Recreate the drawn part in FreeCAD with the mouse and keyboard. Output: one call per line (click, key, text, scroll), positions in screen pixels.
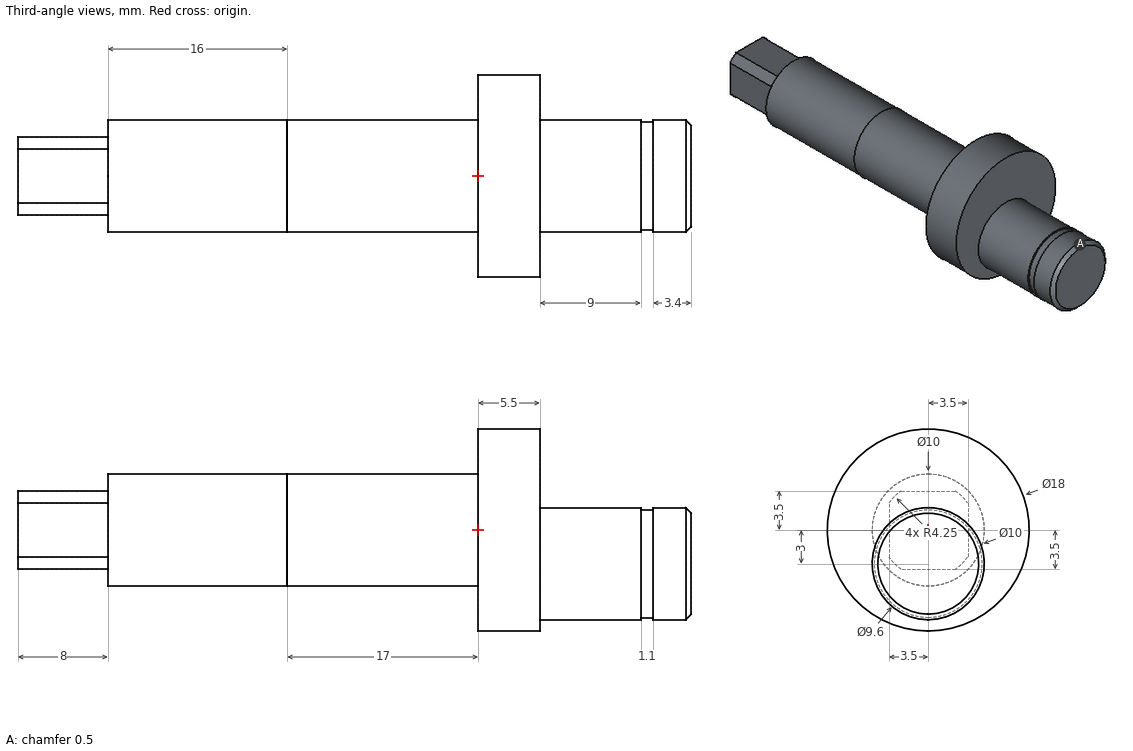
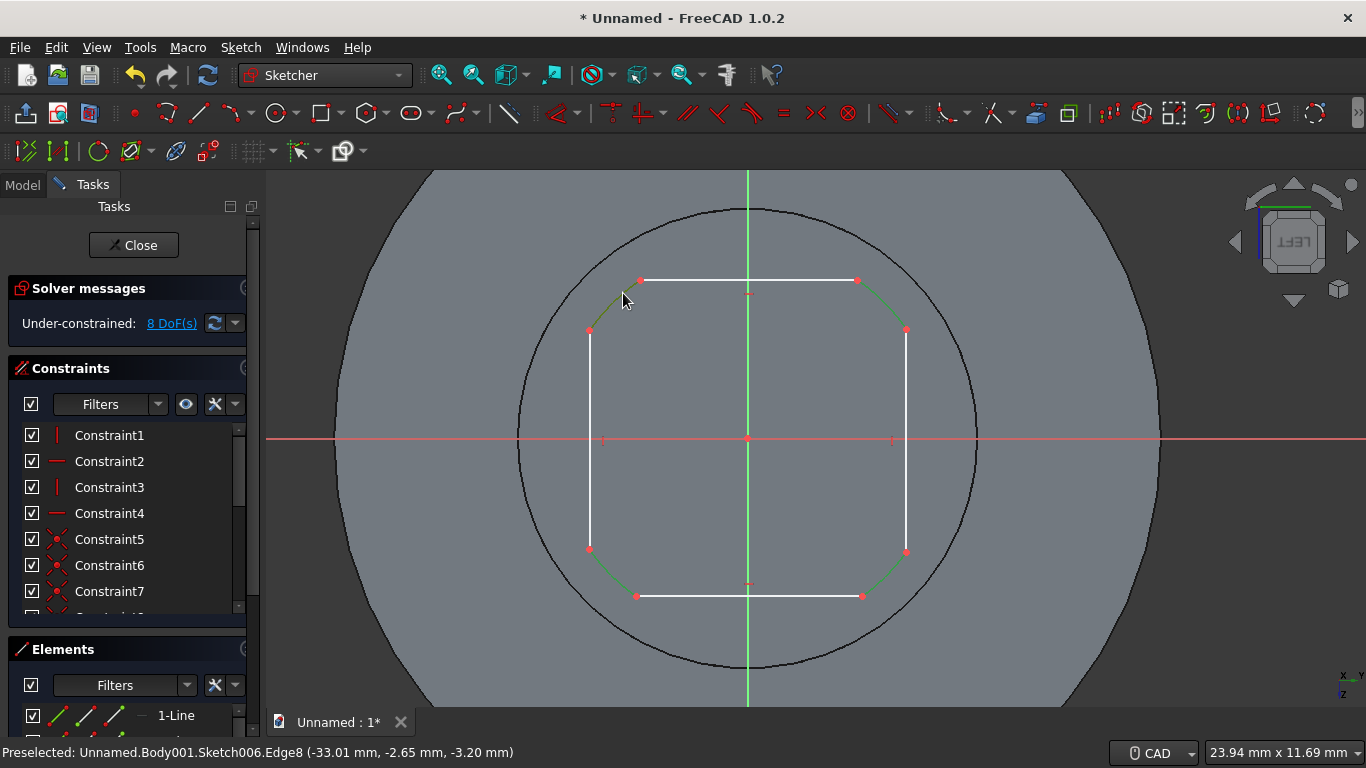
click(784, 114)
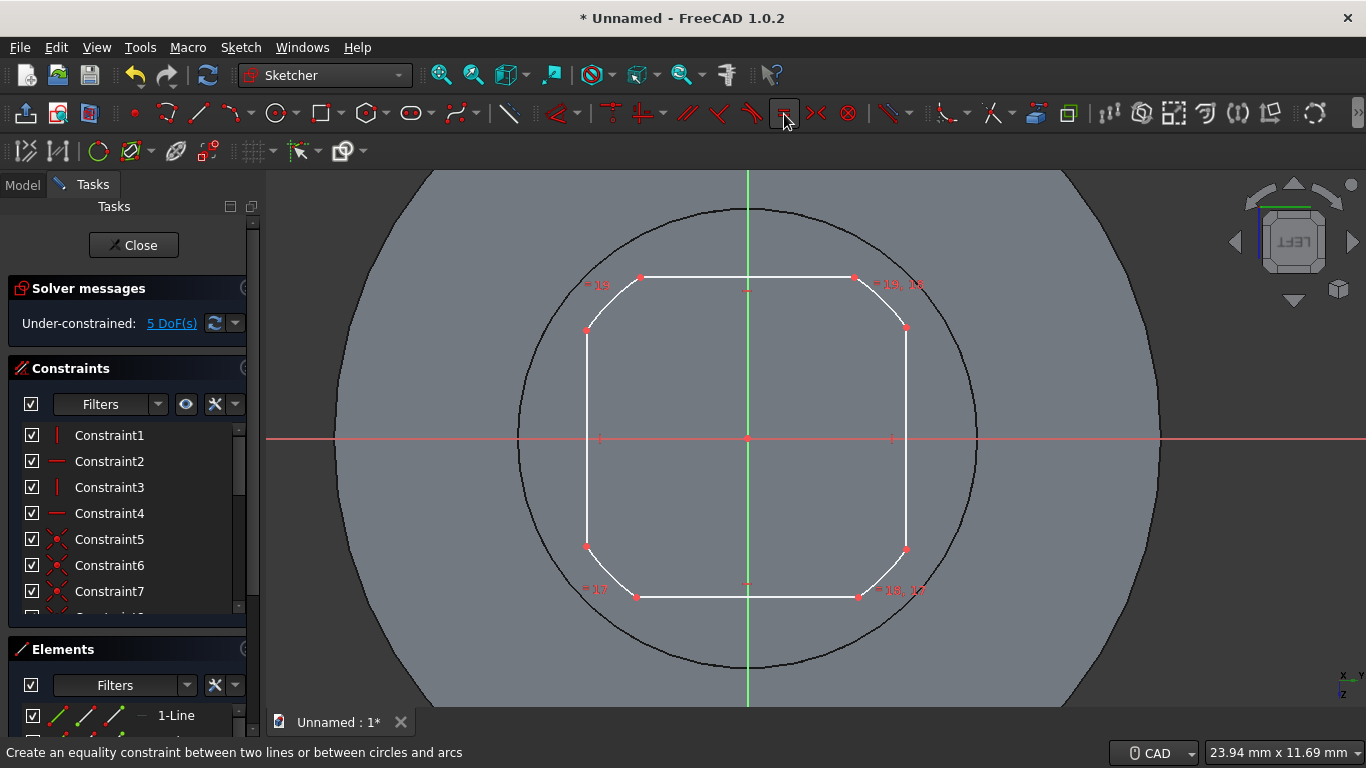
key(d)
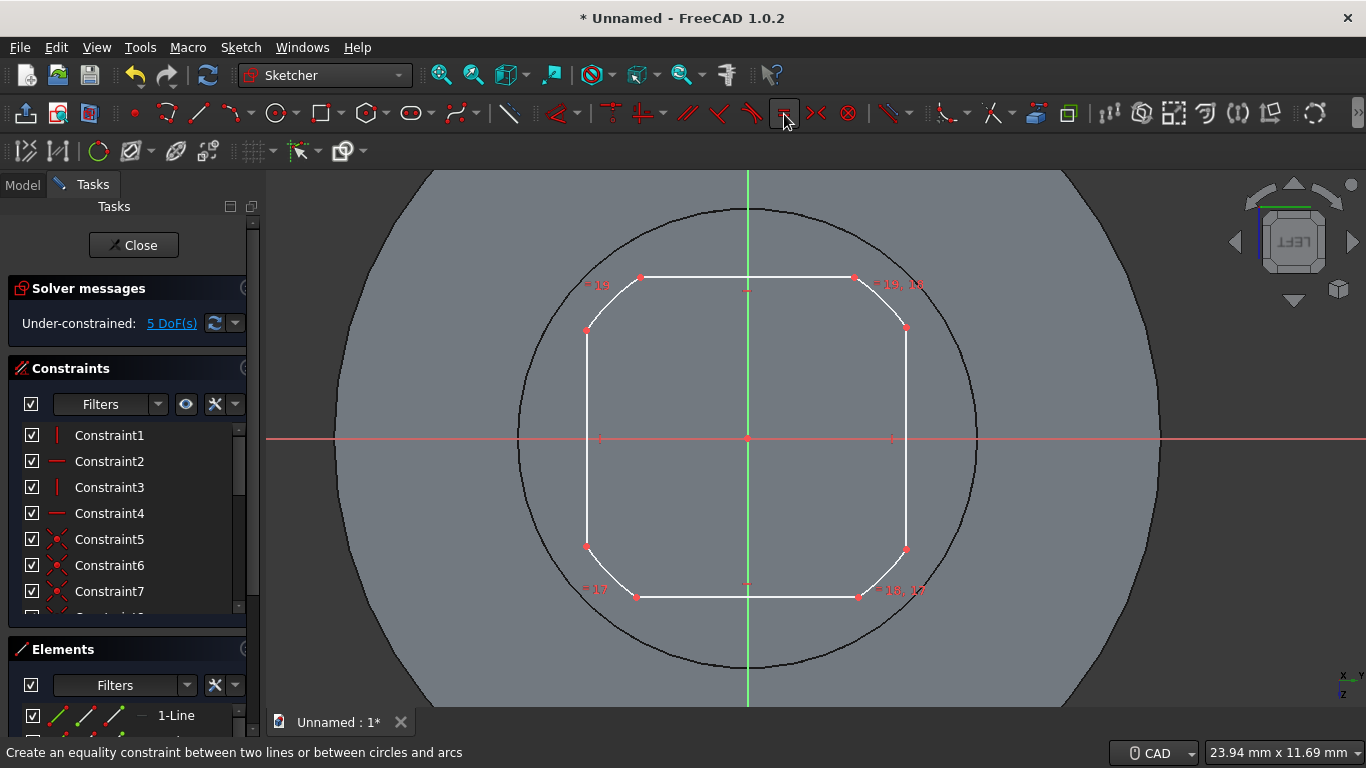
click(600, 563)
click(576, 584)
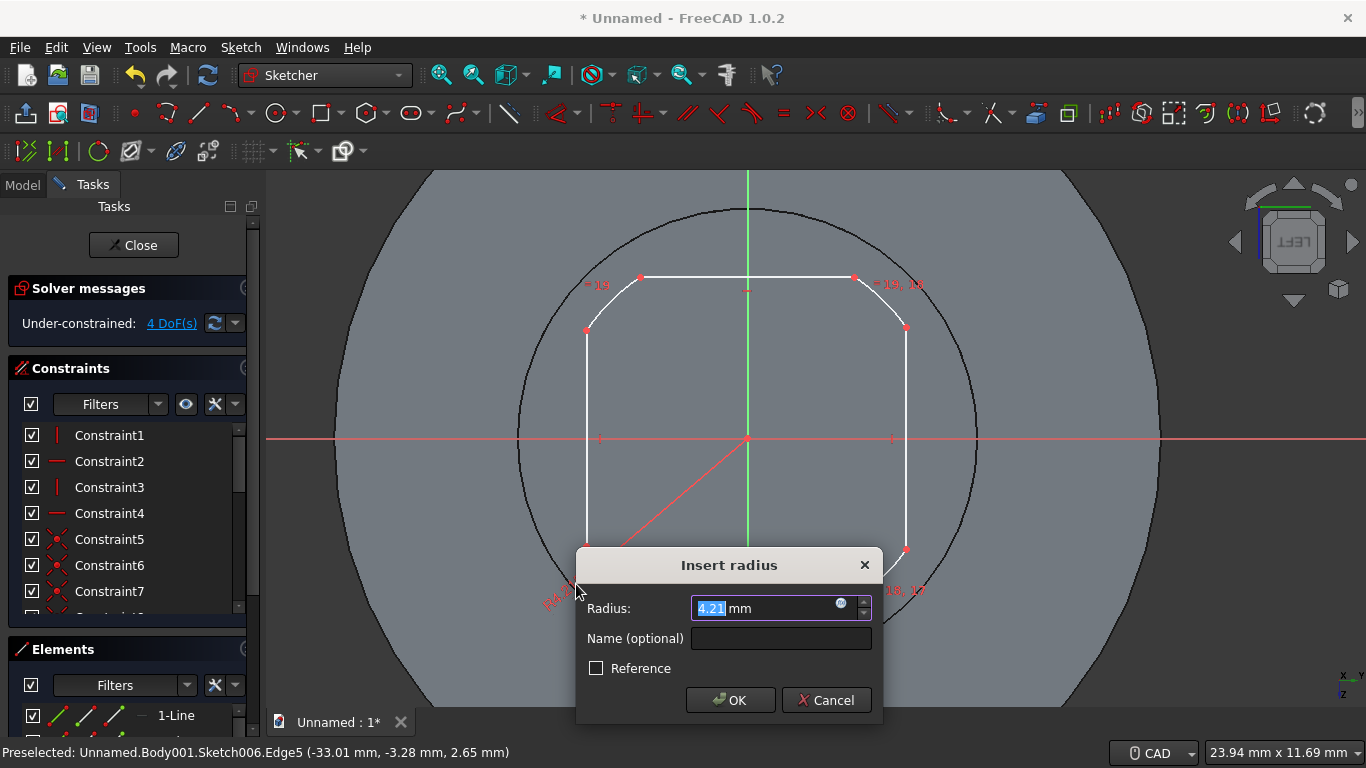
text(4.25)
key(Return)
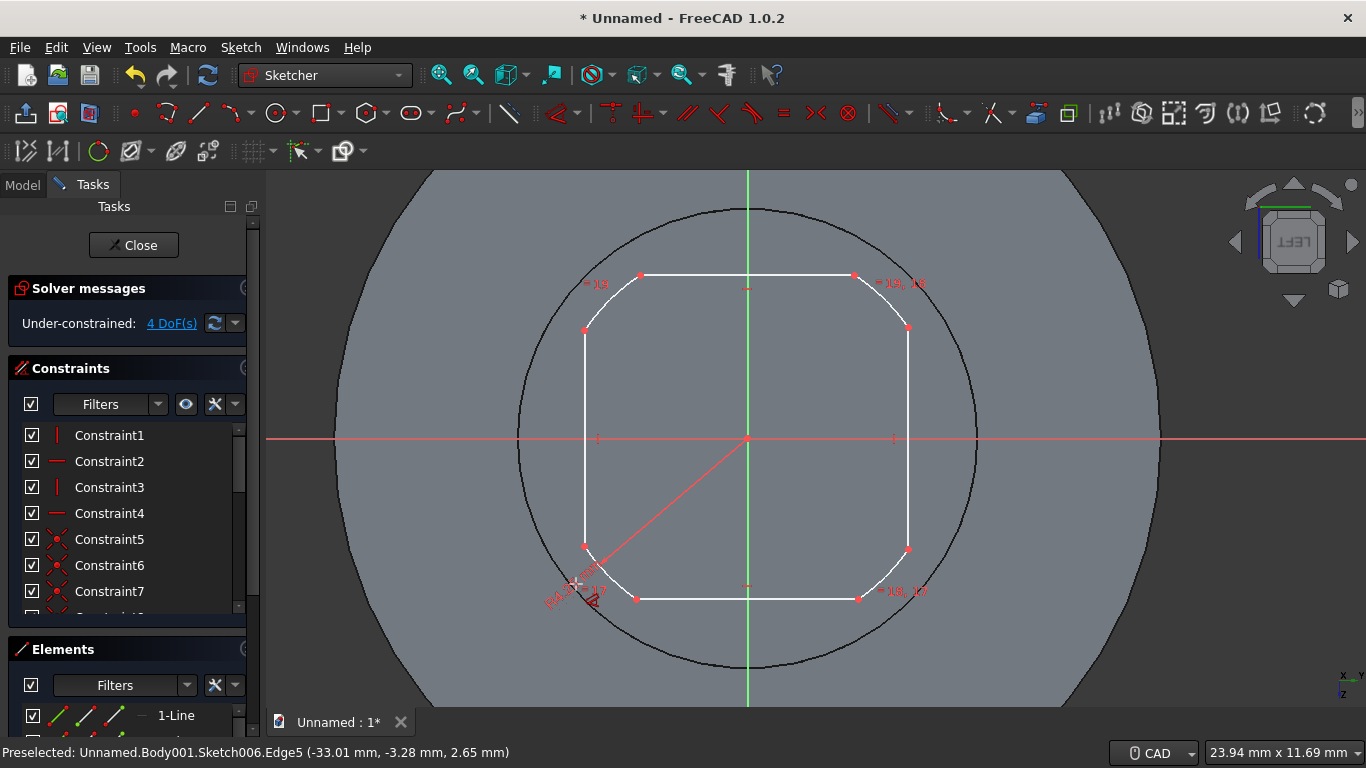
click(585, 331)
click(666, 297)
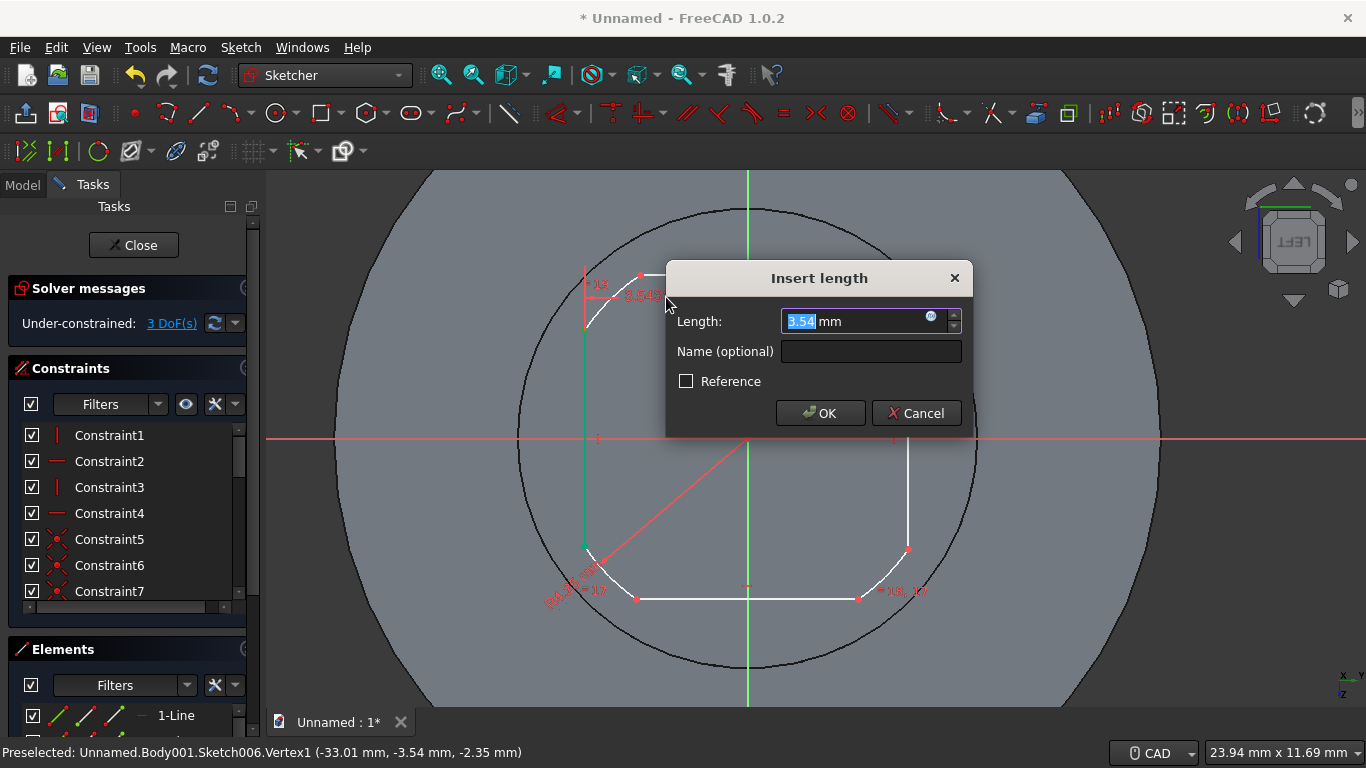
text(3.5)
key(Return)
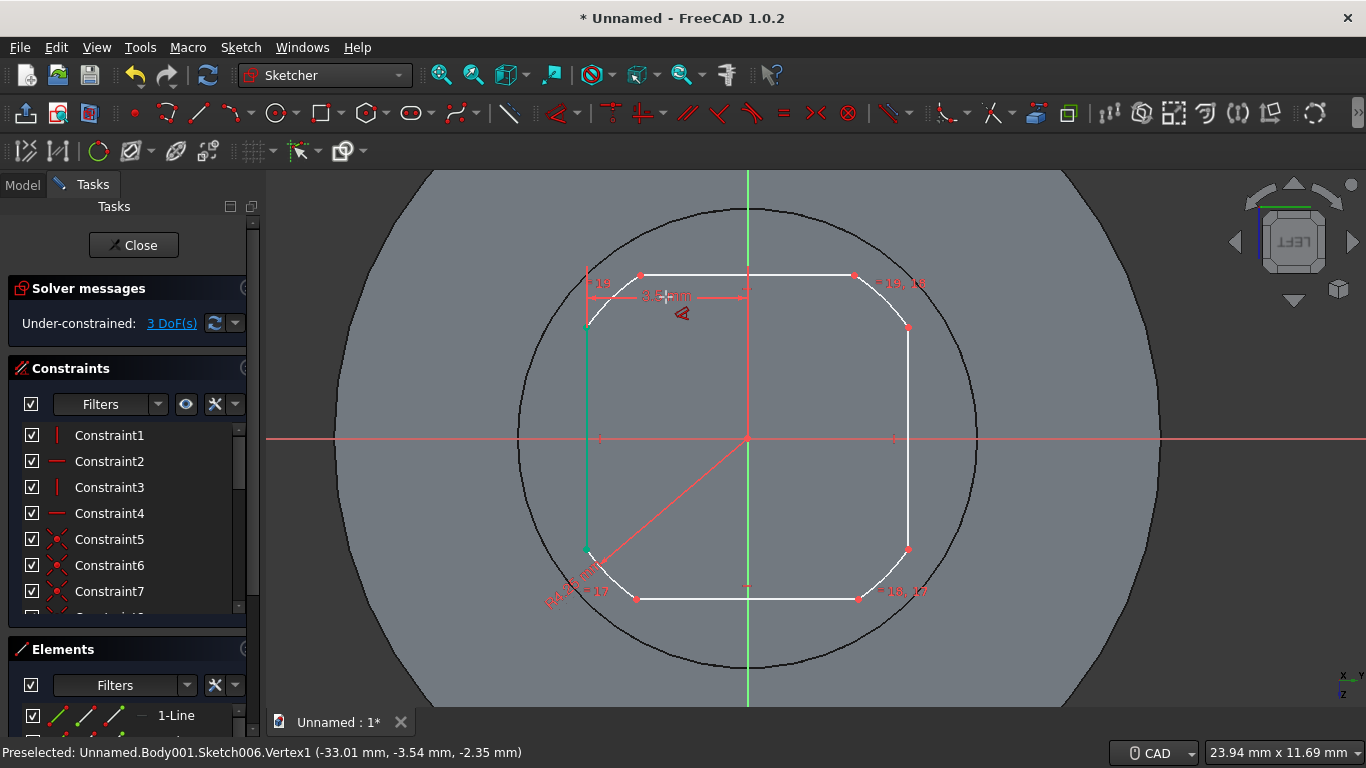
click(636, 599)
click(602, 519)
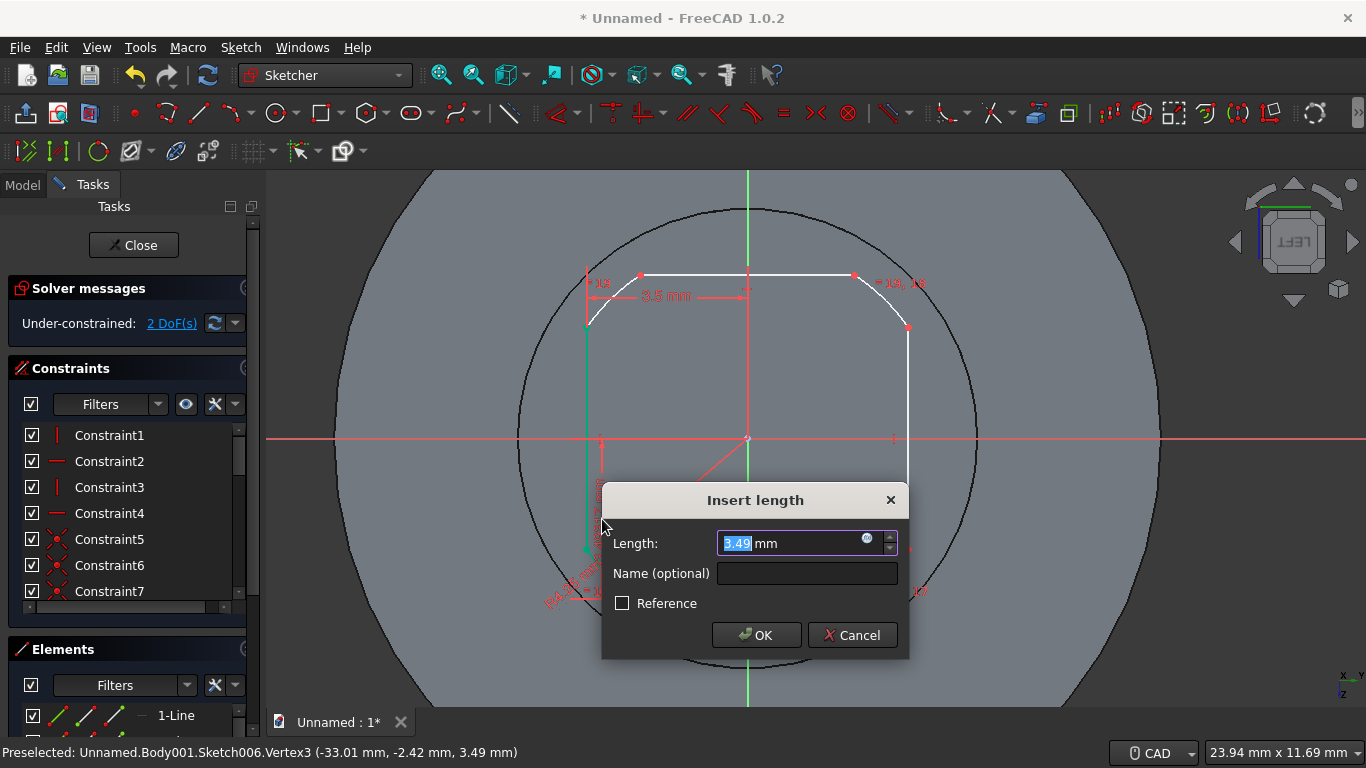
text(3.5)
key(Return)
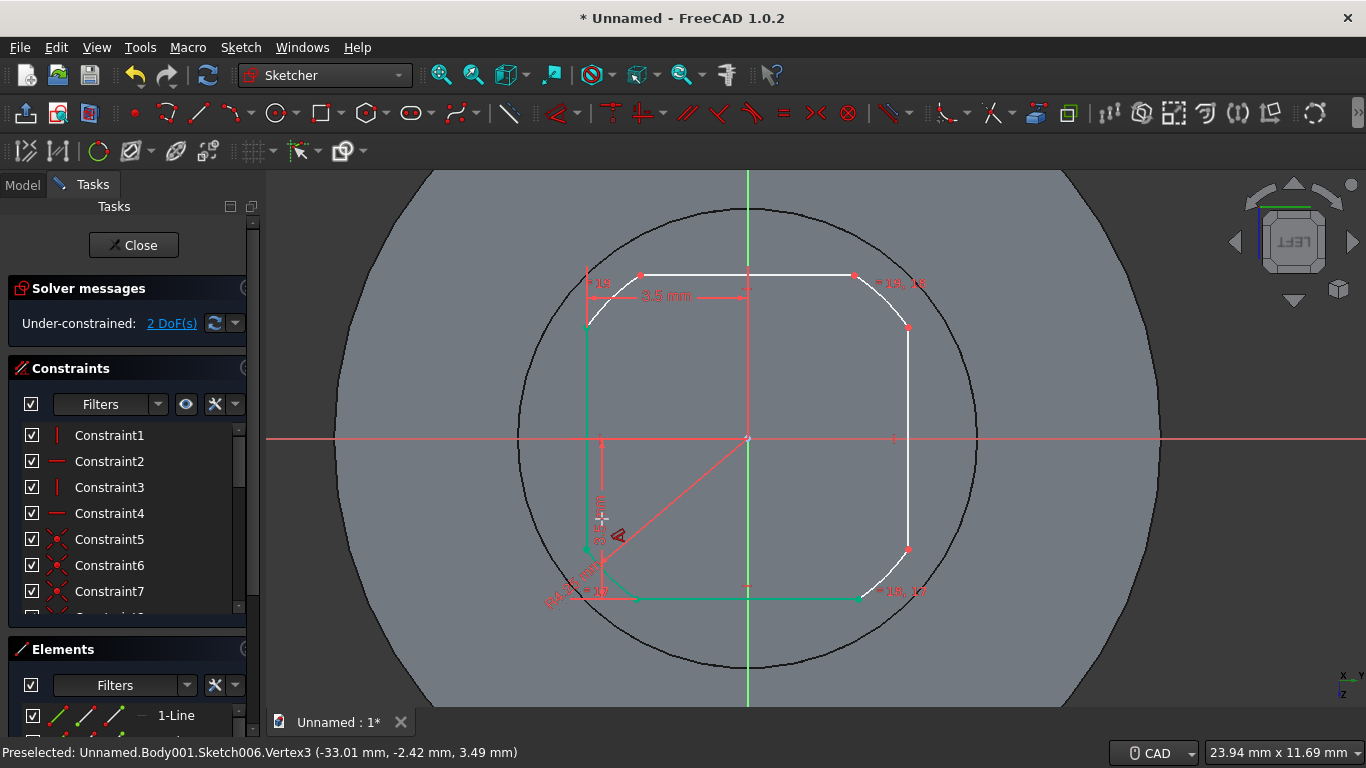
click(908, 549)
click(828, 583)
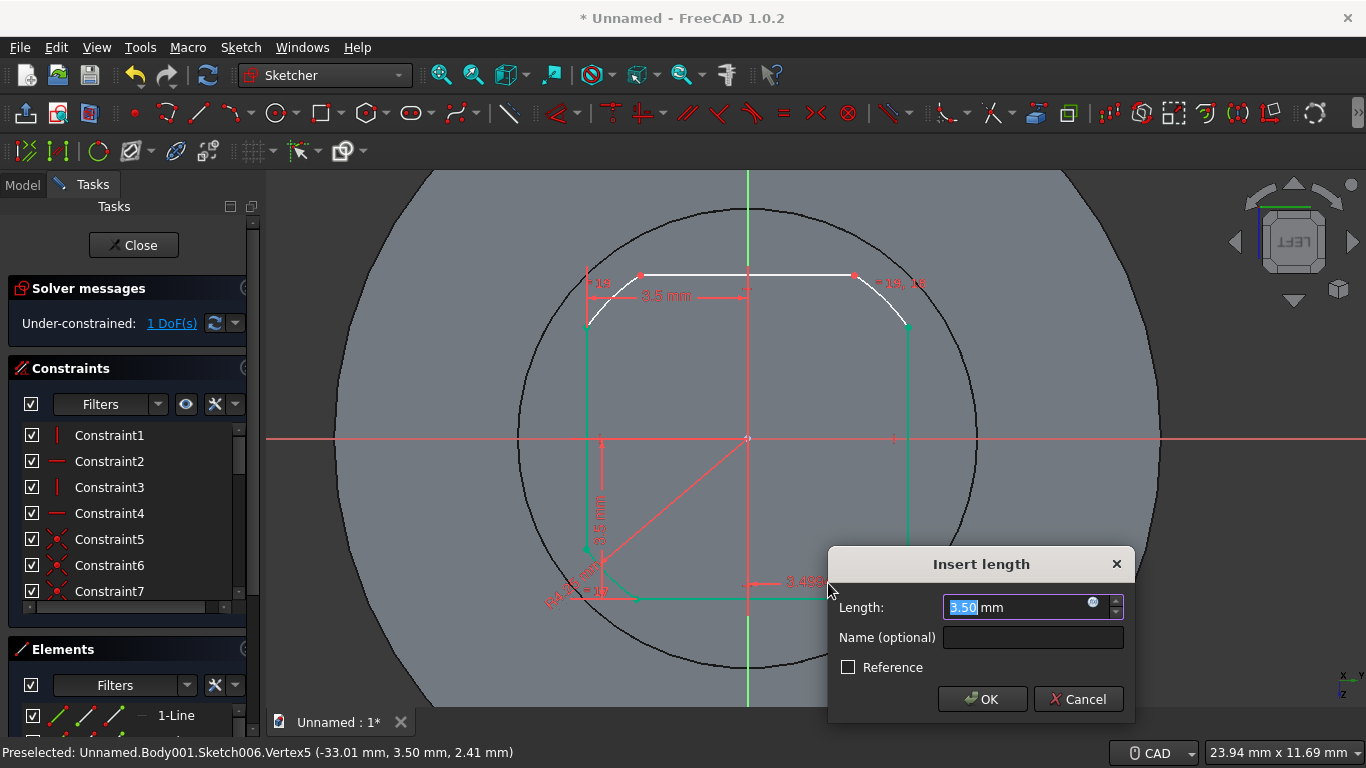
text(3.5)
key(Return)